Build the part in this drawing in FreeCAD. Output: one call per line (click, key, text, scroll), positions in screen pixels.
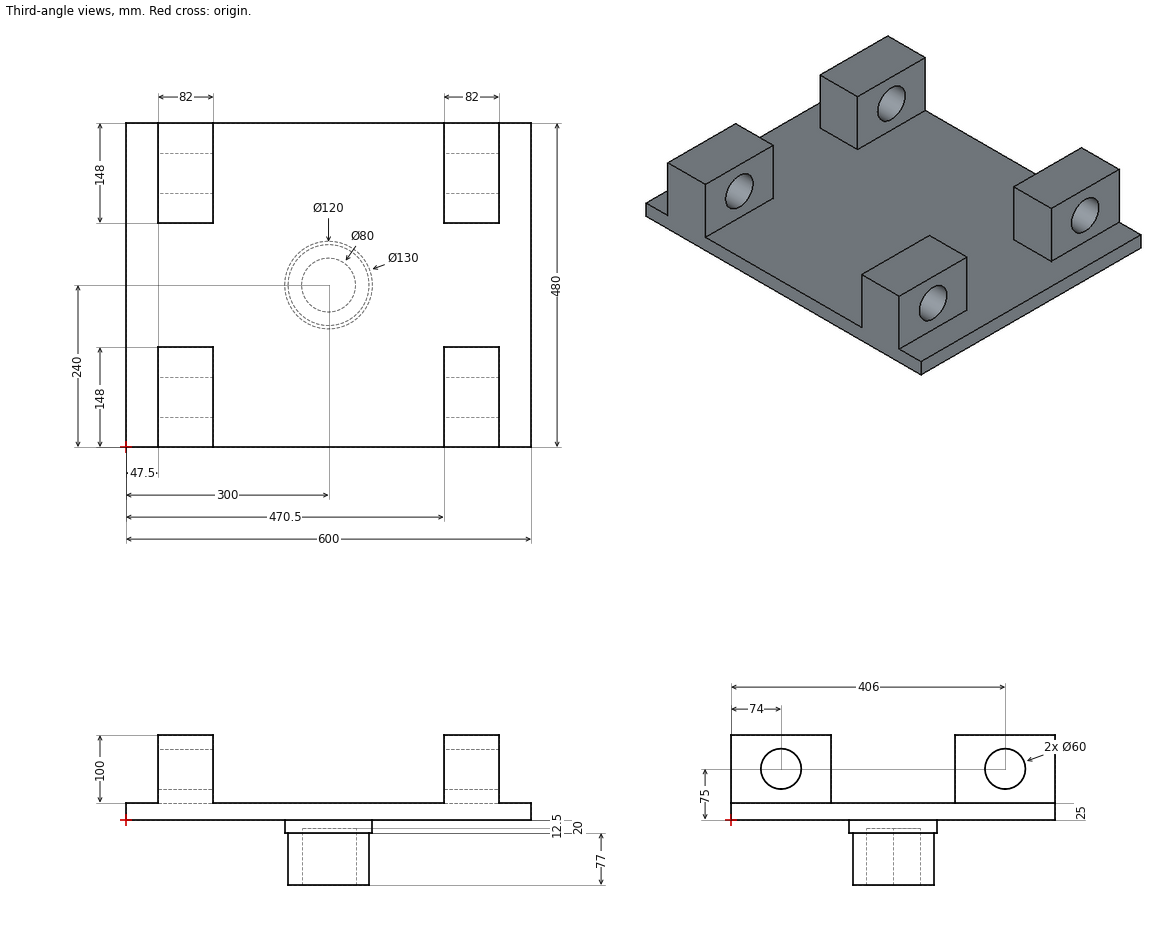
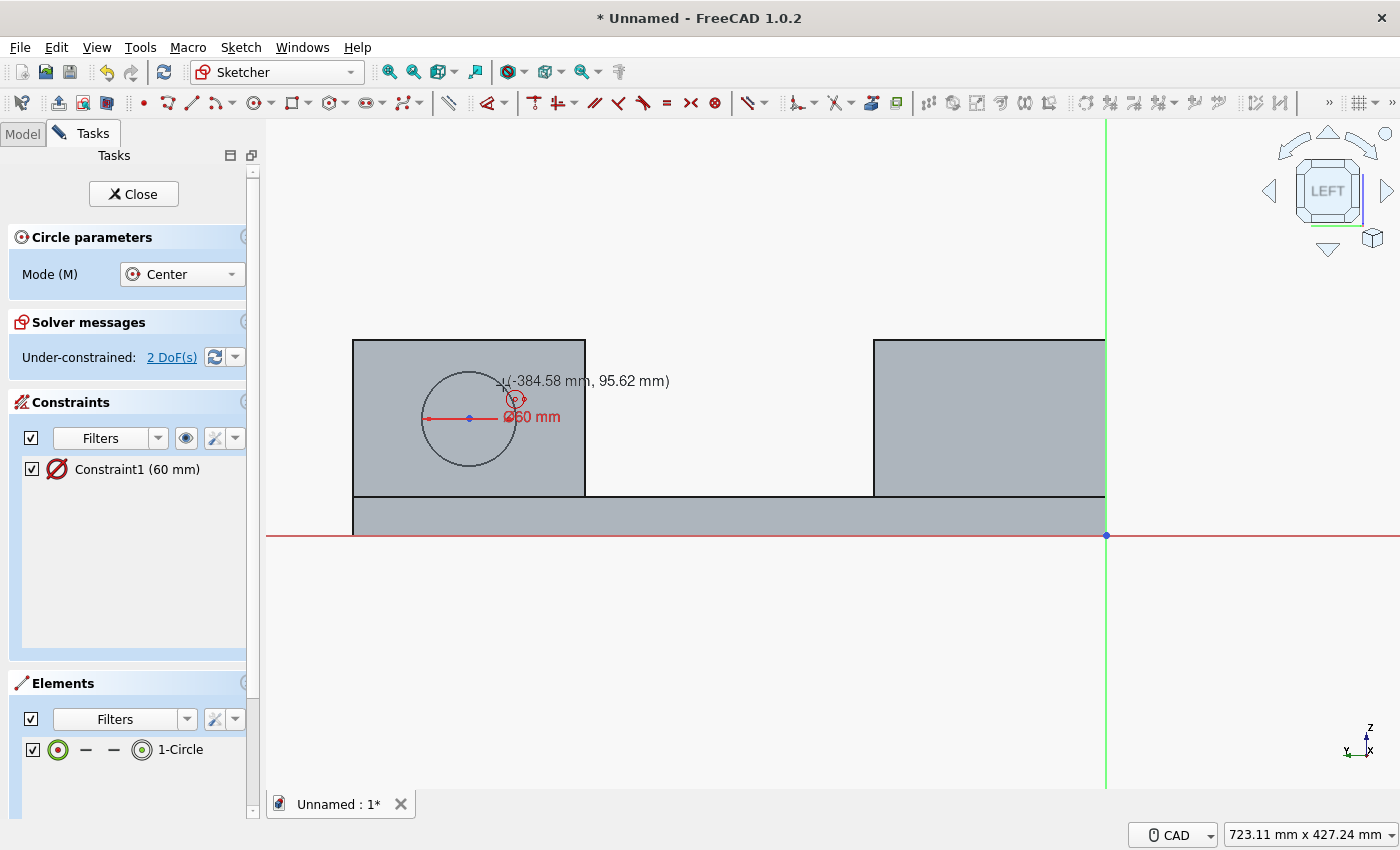
click(990, 418)
move(1023, 385)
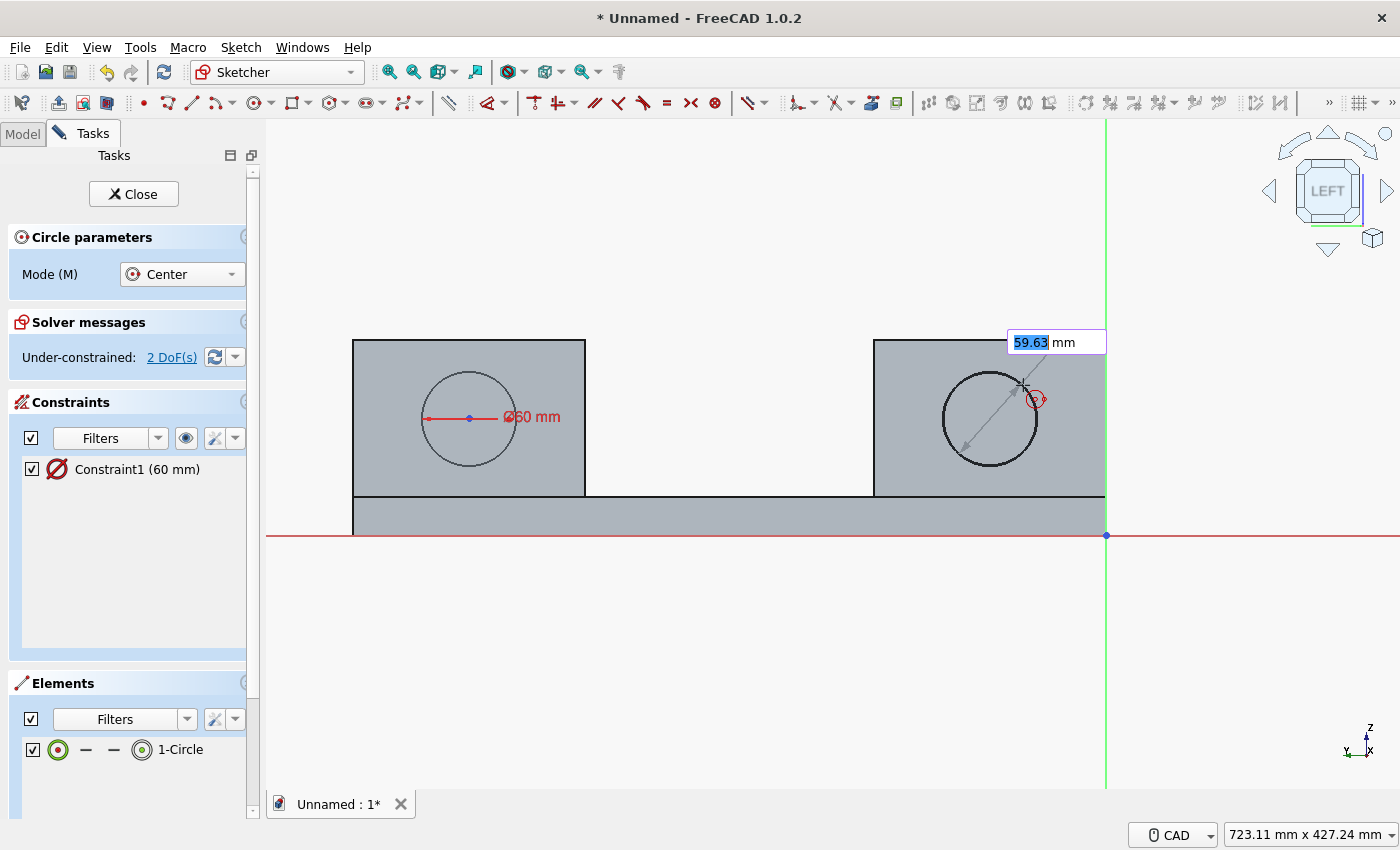
text(60)
key(Return)
key(Escape)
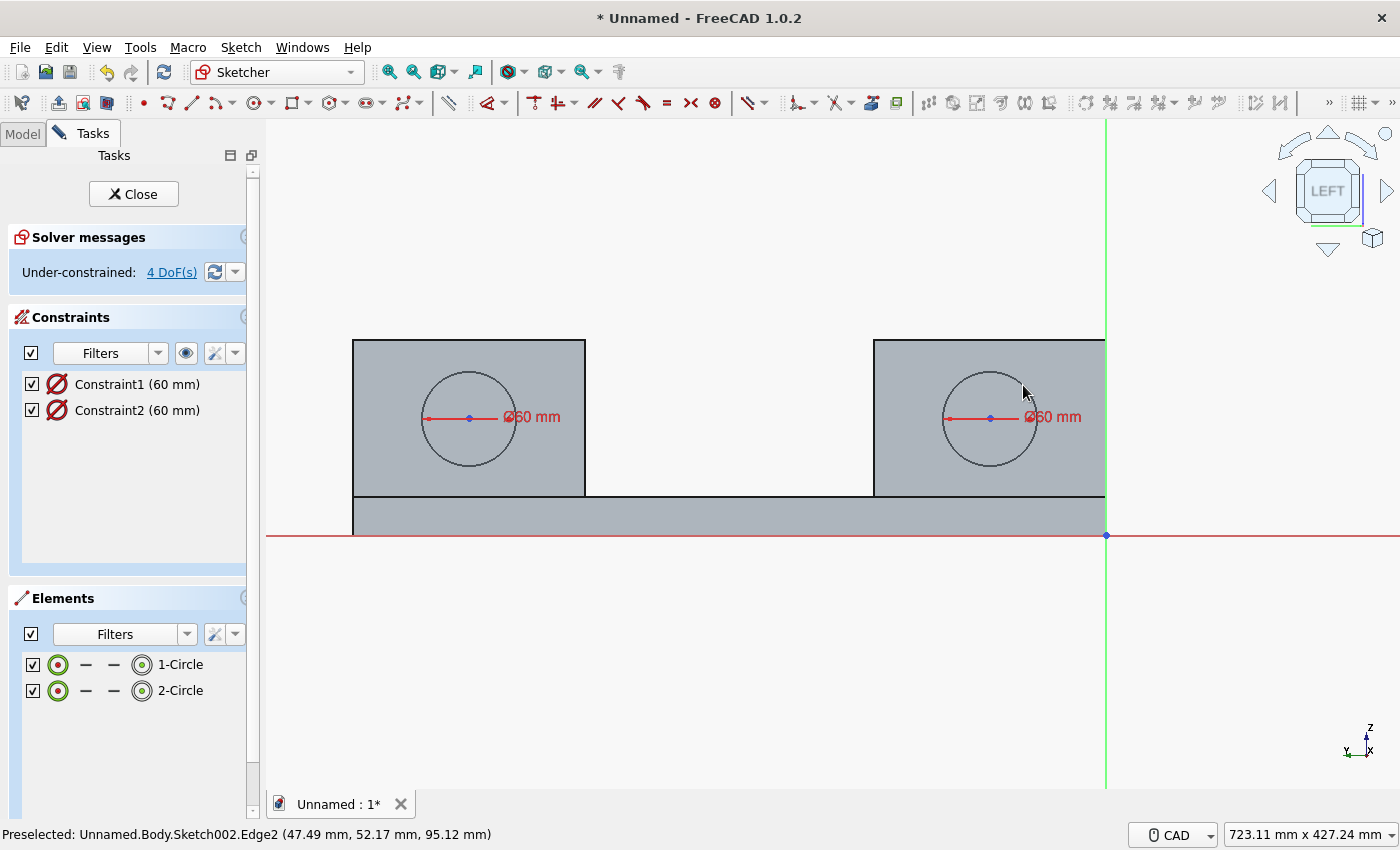
click(469, 419)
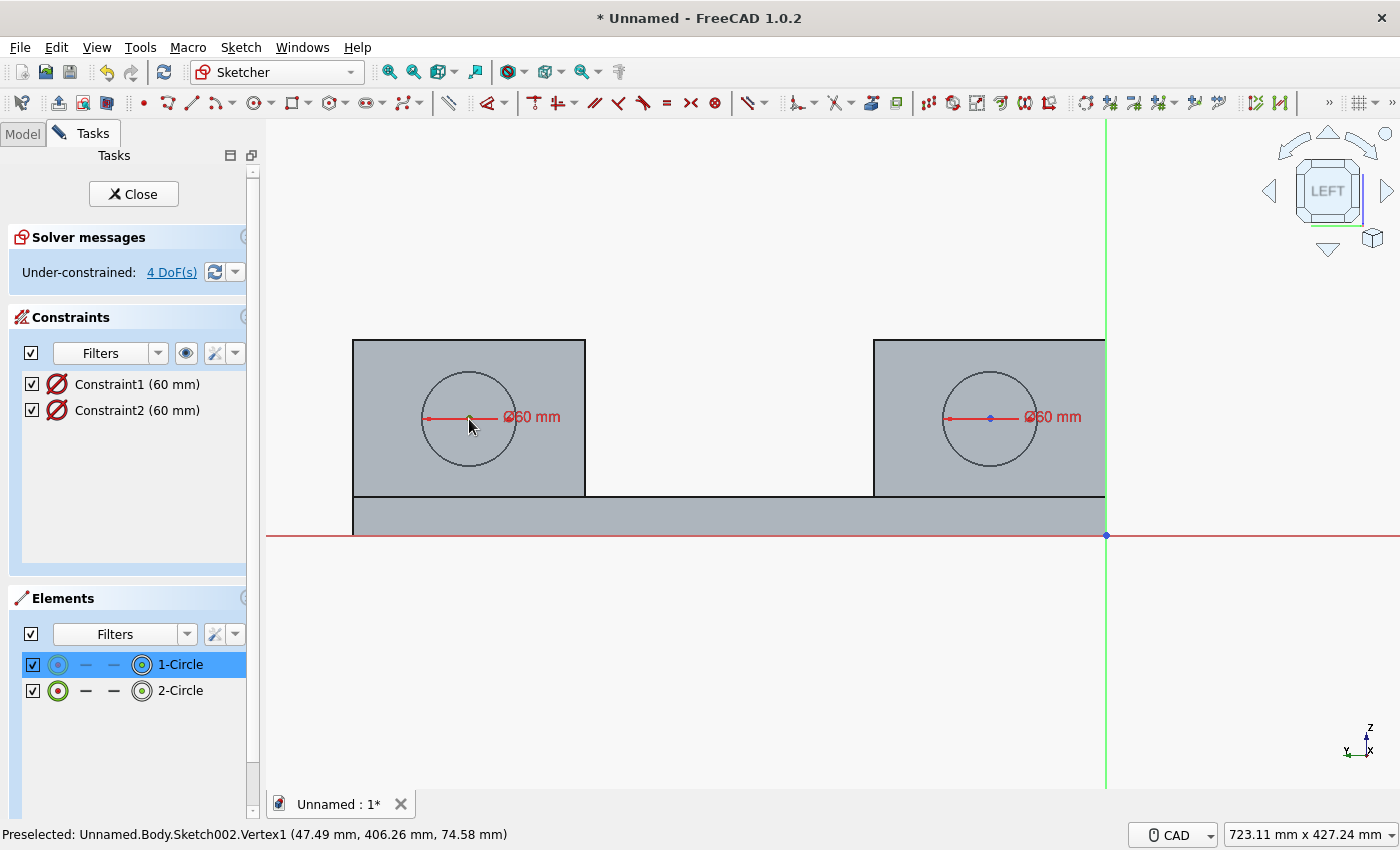
click(990, 419)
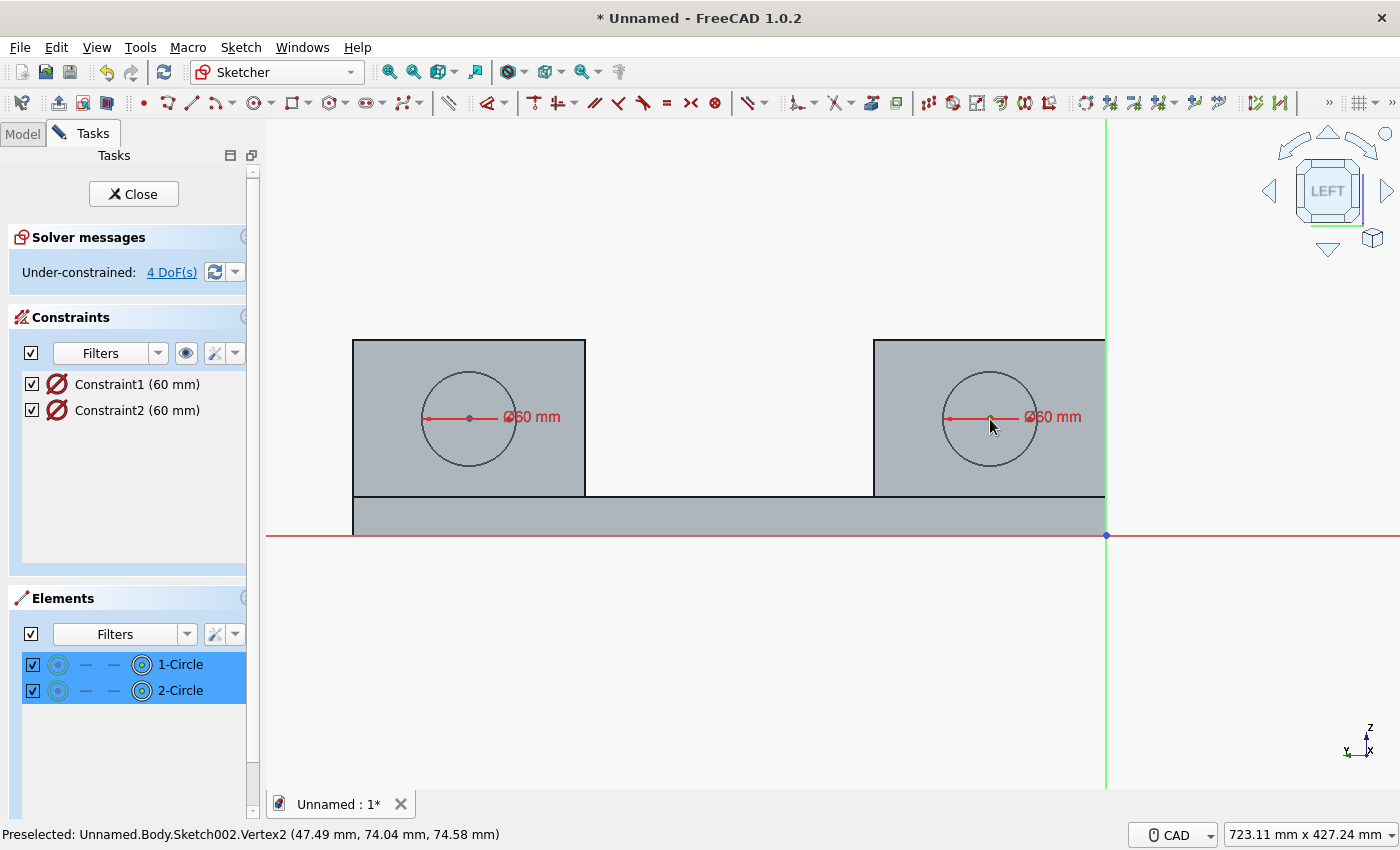
click(576, 104)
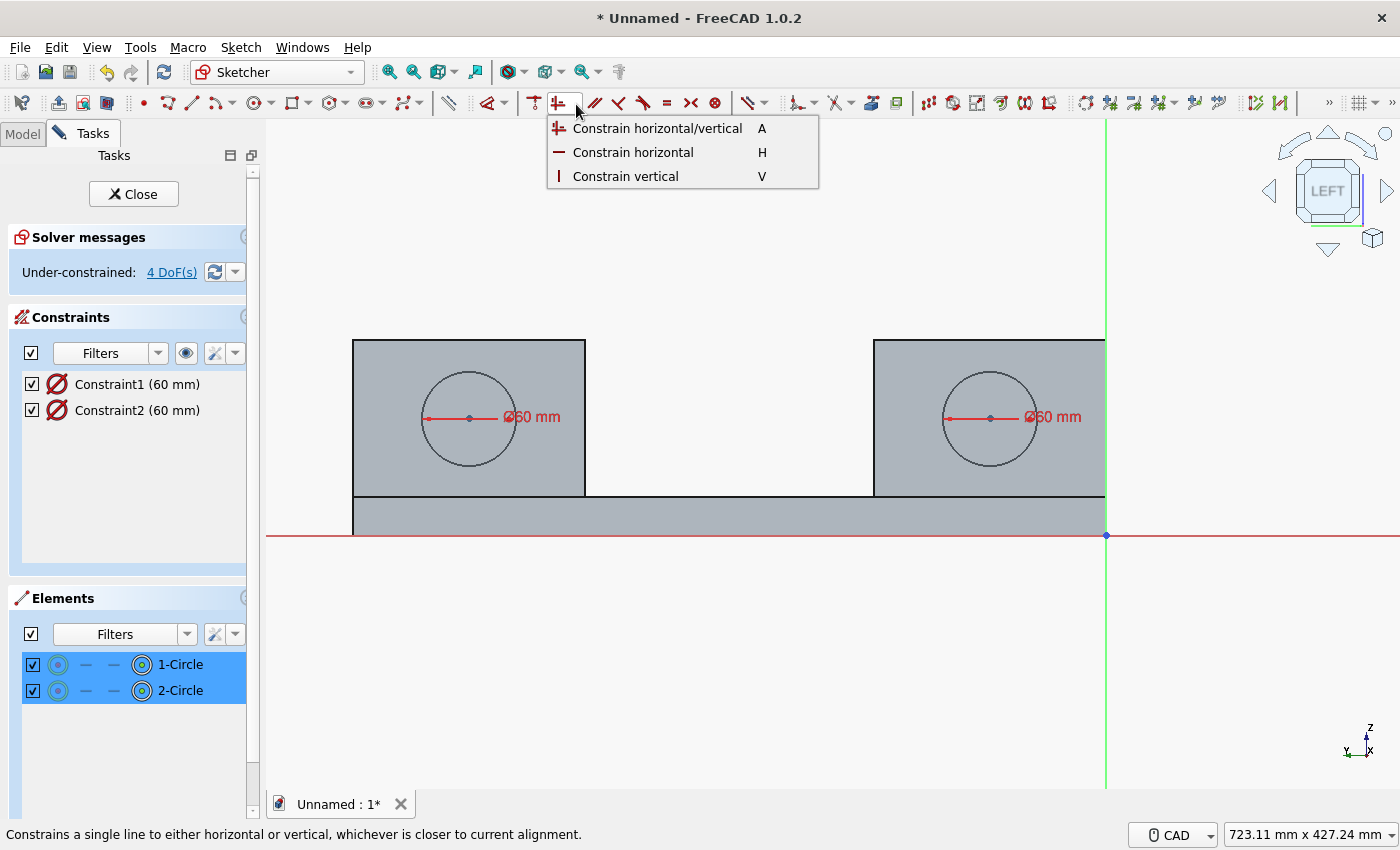
click(683, 152)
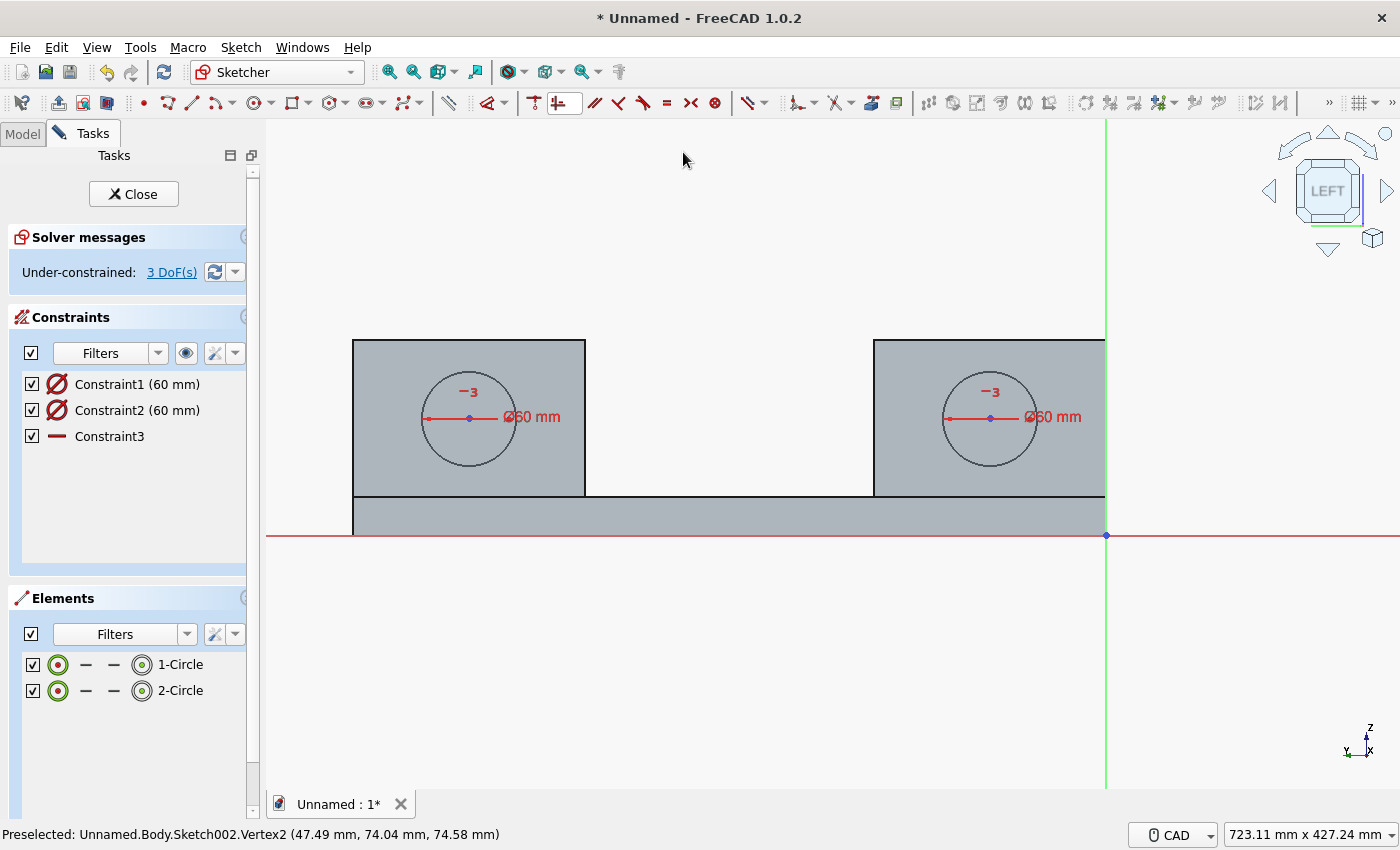
click(488, 104)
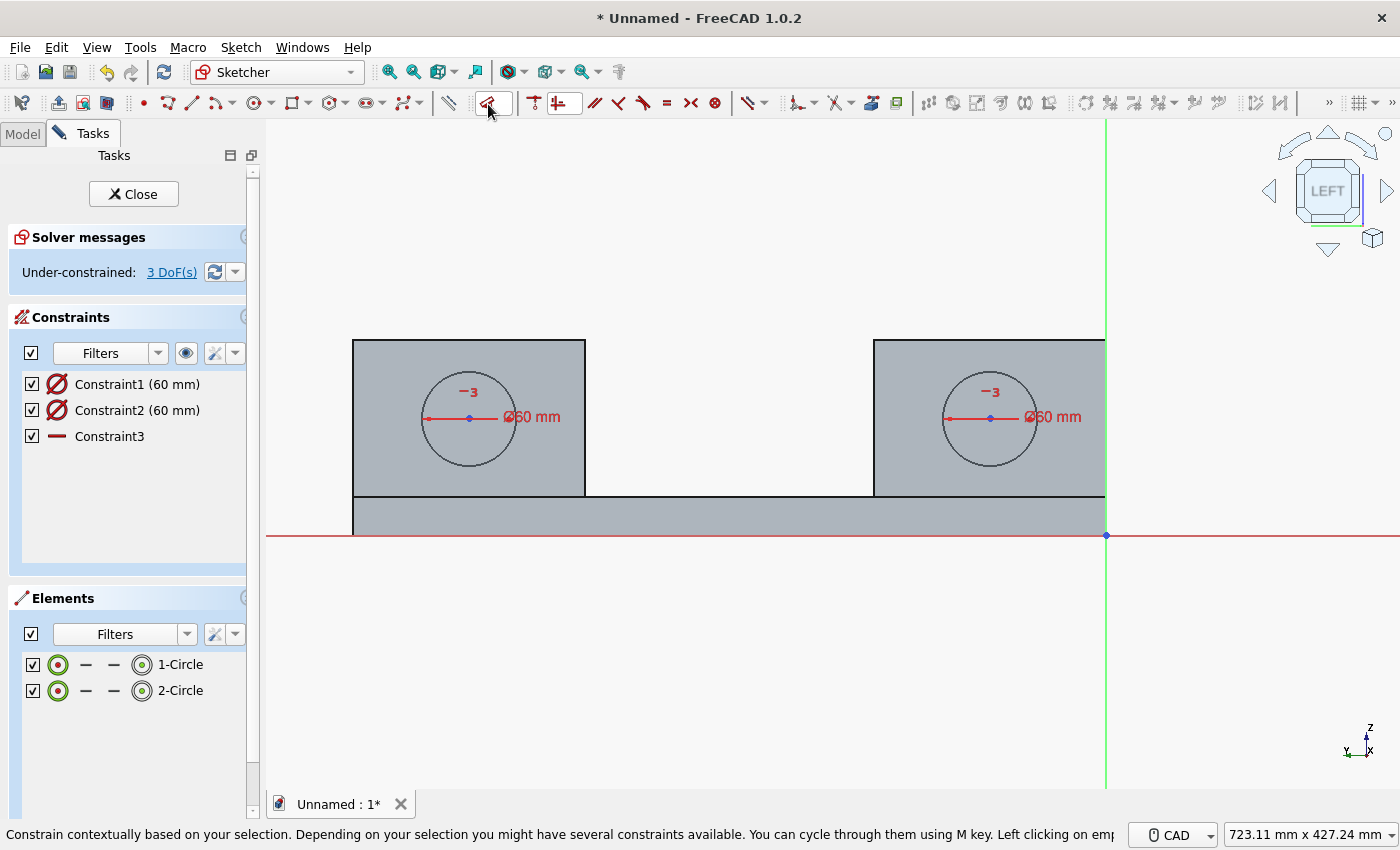
click(469, 419)
click(1140, 477)